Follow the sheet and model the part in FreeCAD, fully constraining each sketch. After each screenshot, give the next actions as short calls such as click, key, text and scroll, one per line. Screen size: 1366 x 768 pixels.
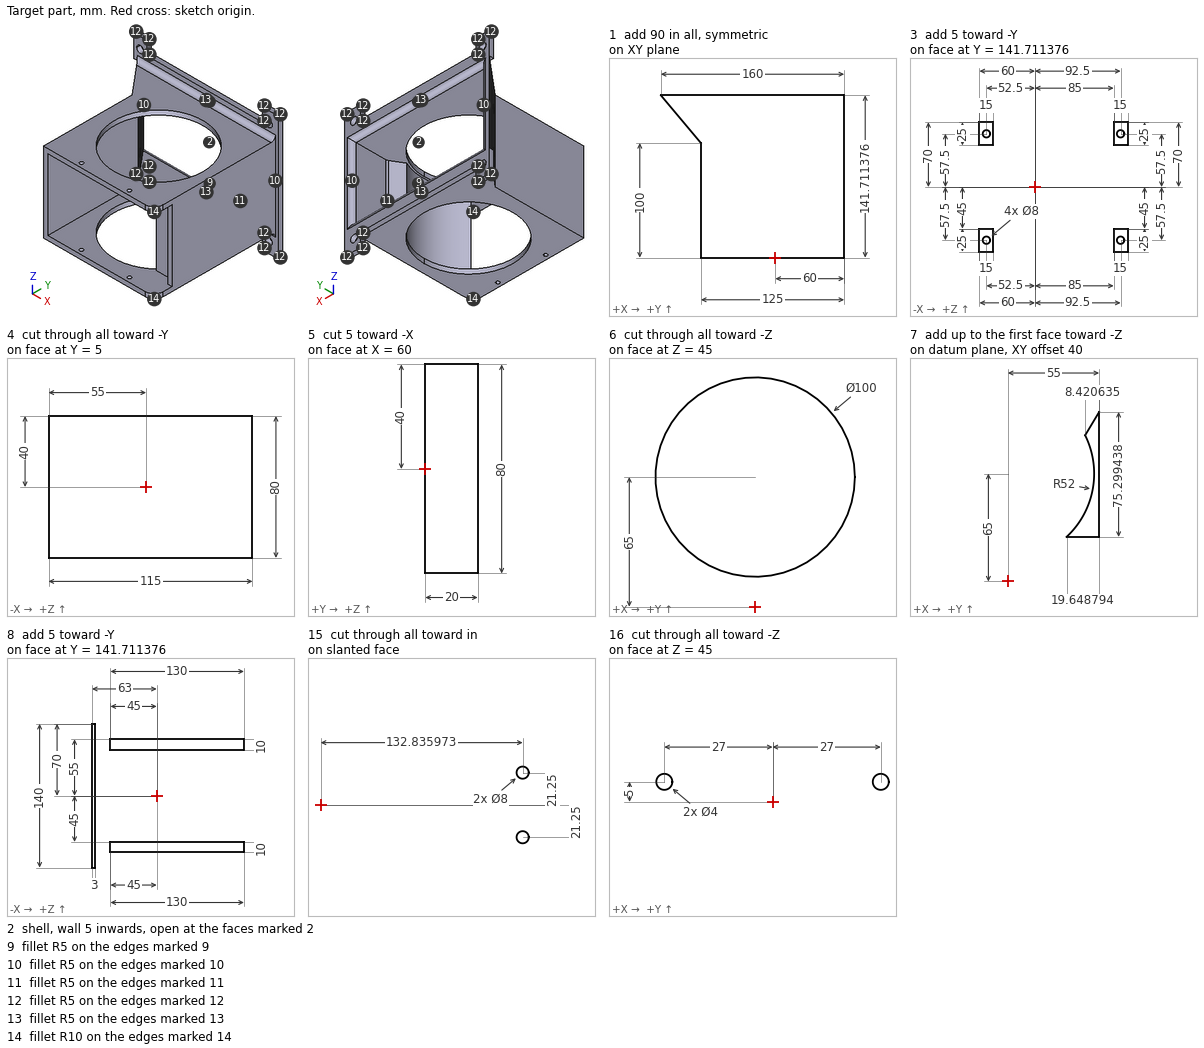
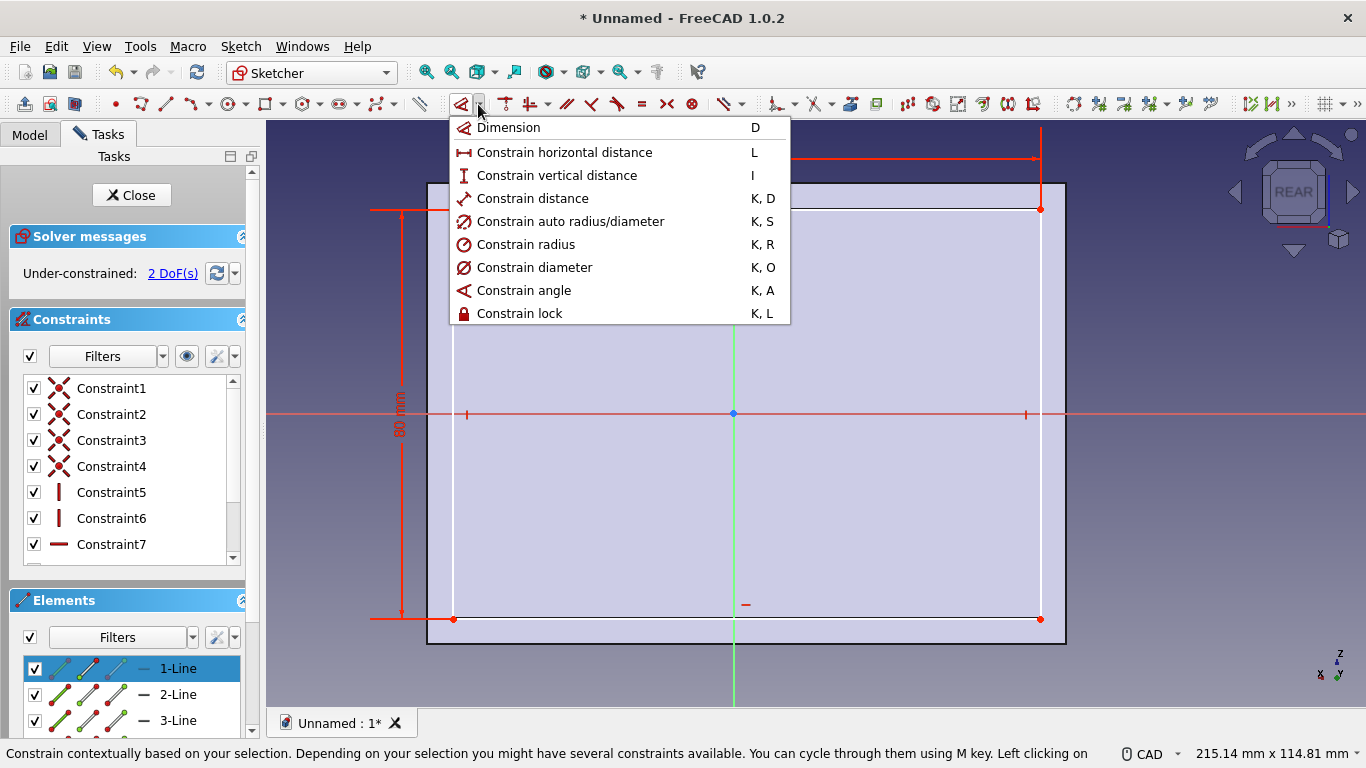
click(620, 152)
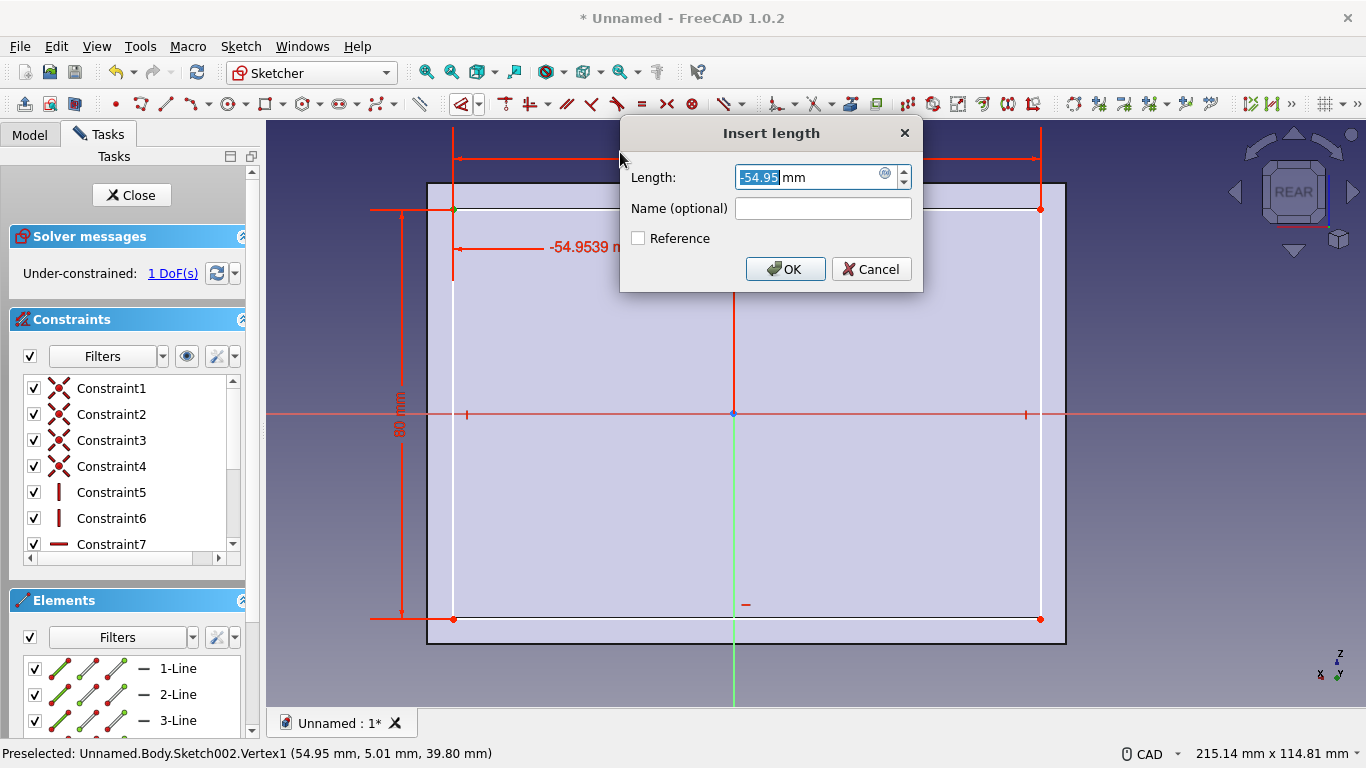
text(-55)
key(Return)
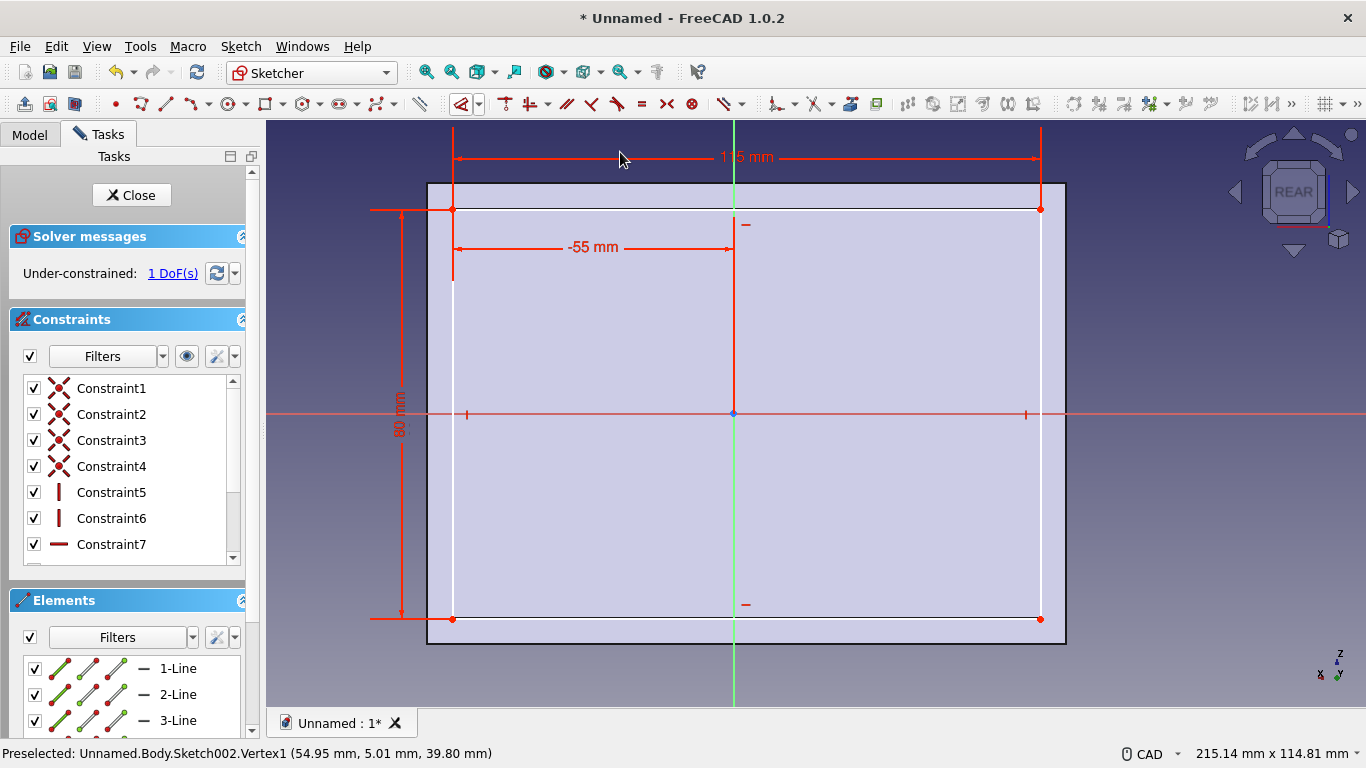
click(453, 210)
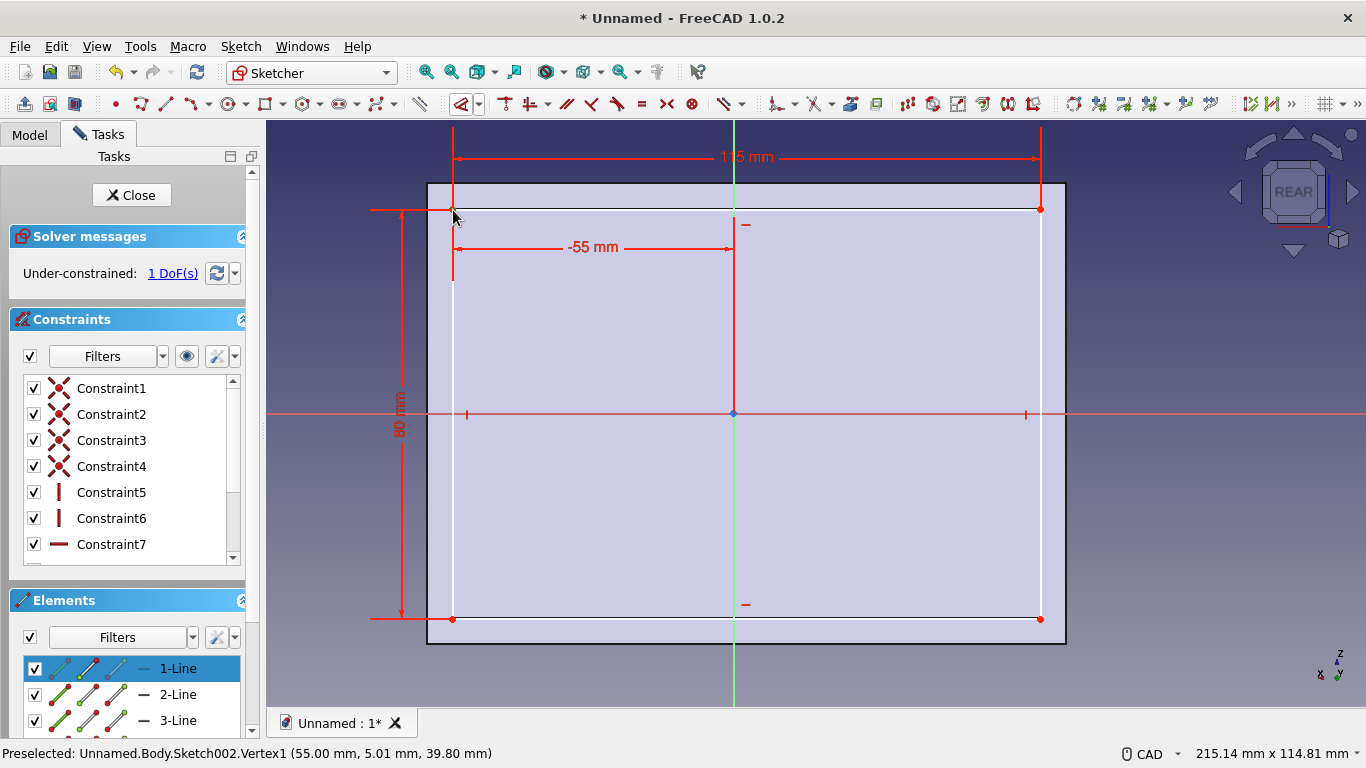
key(i)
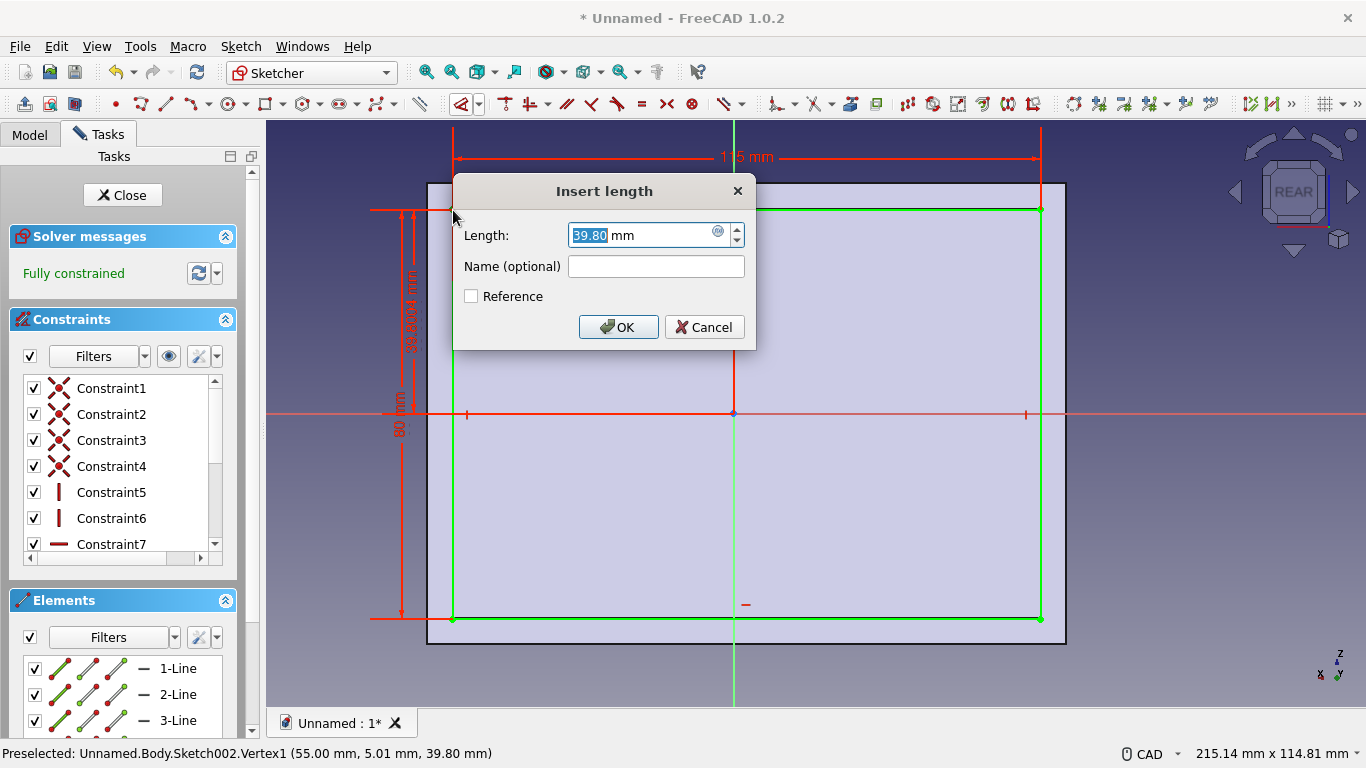
text(40)
key(Return)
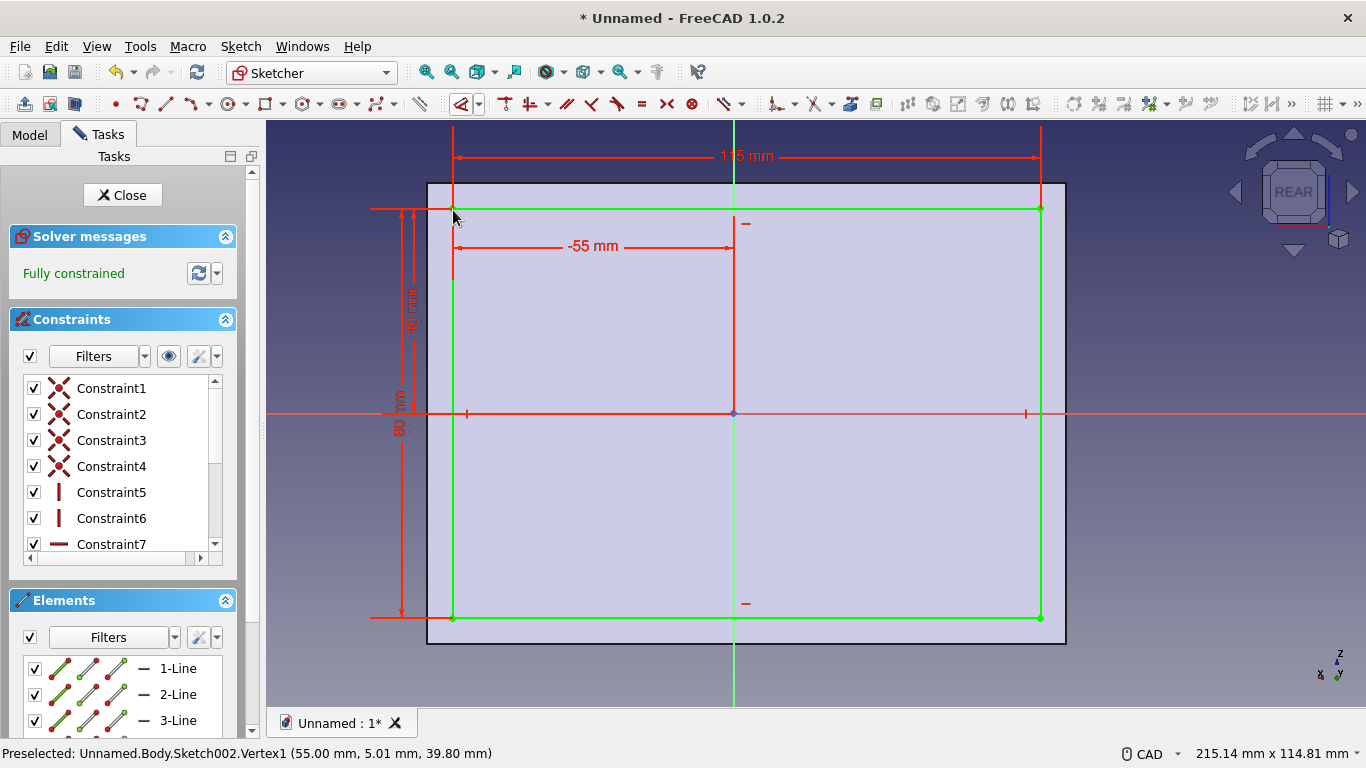
click(123, 195)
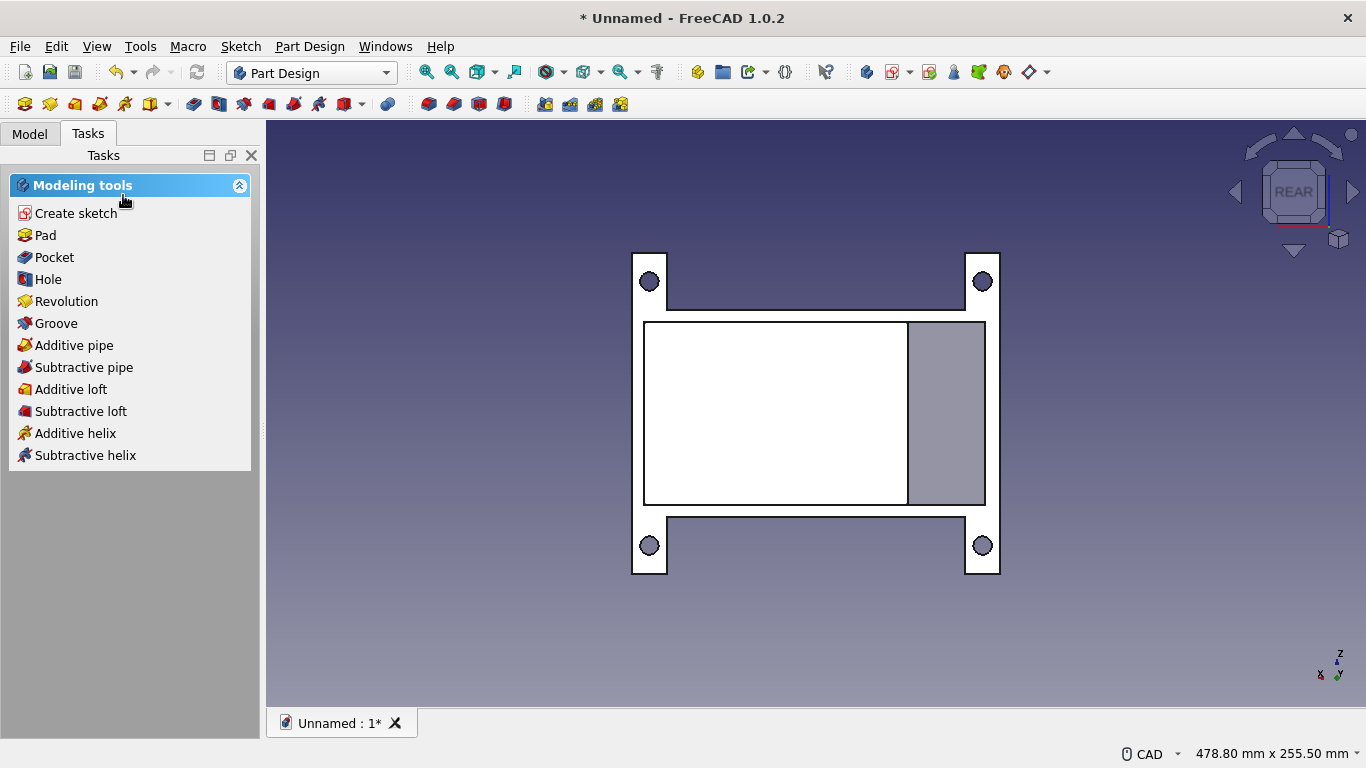
click(194, 104)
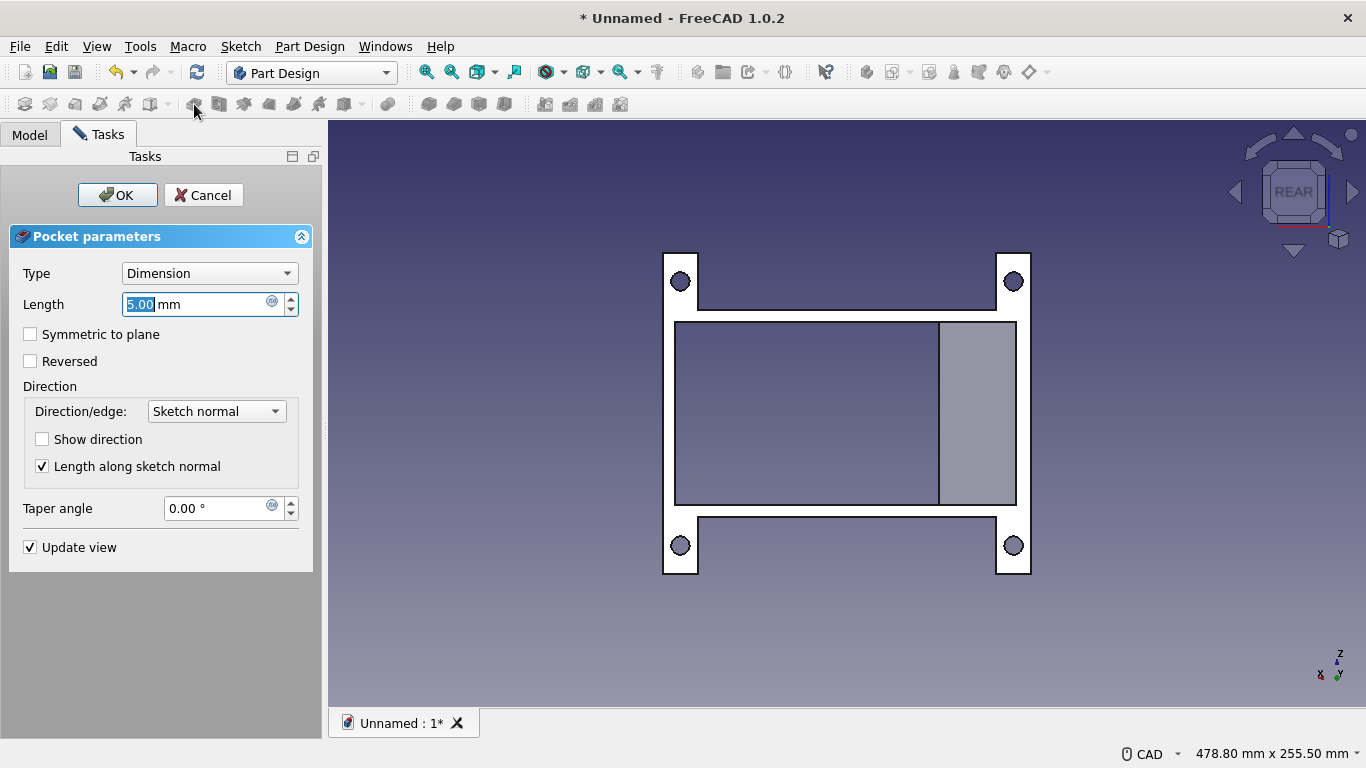
click(210, 274)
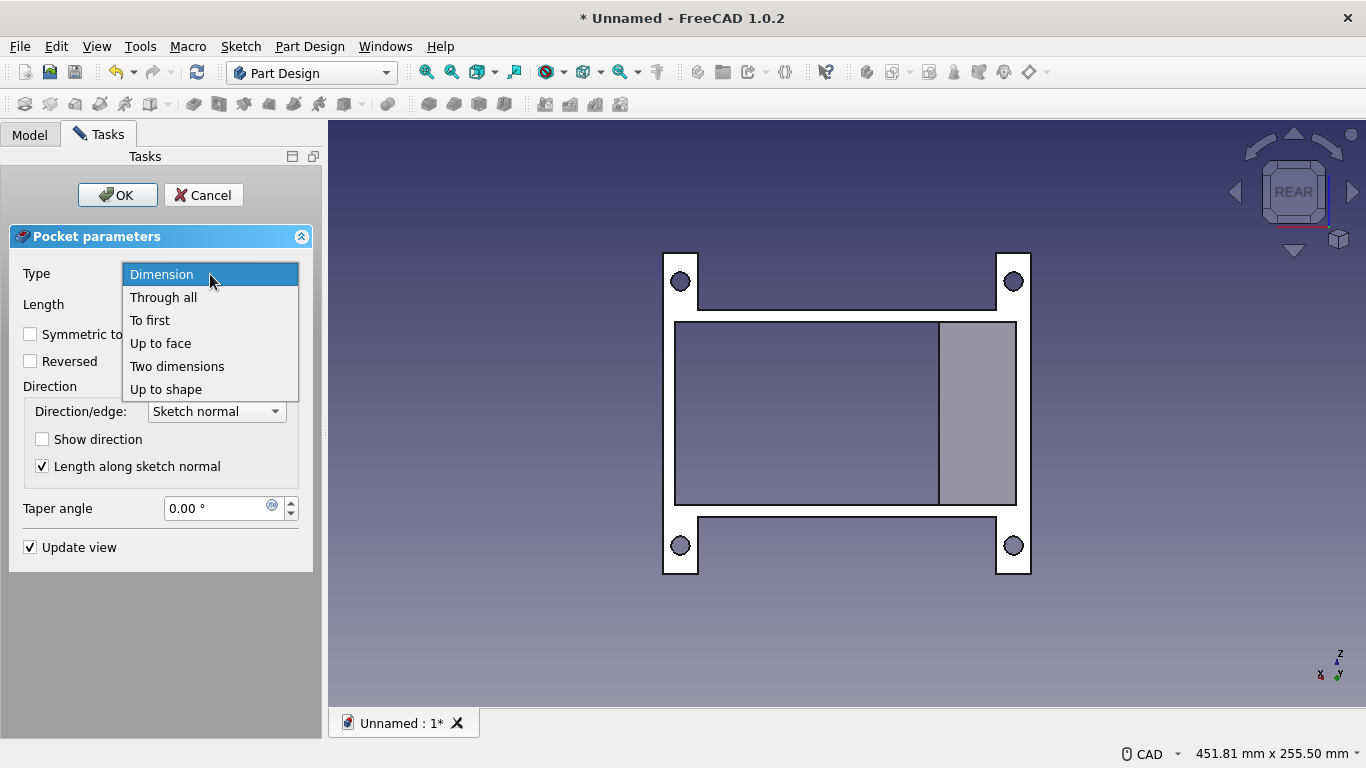
click(208, 298)